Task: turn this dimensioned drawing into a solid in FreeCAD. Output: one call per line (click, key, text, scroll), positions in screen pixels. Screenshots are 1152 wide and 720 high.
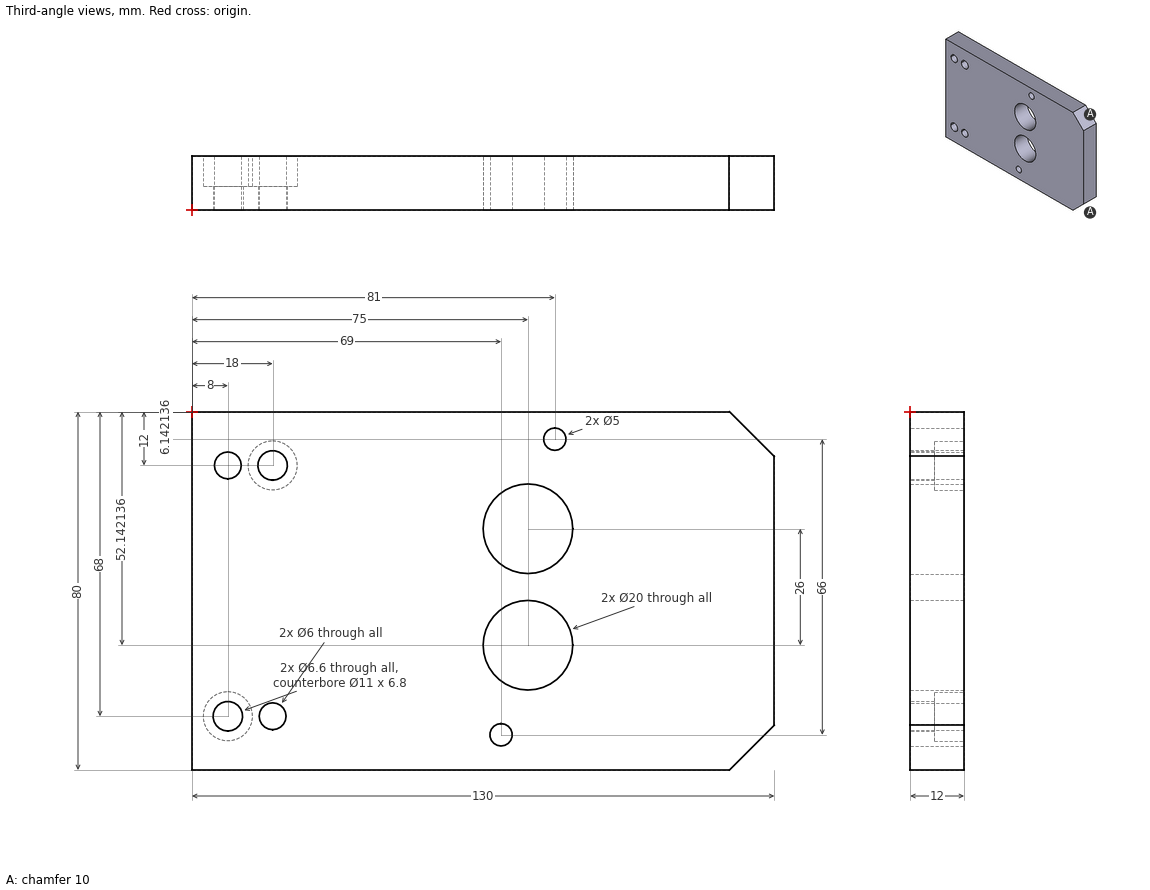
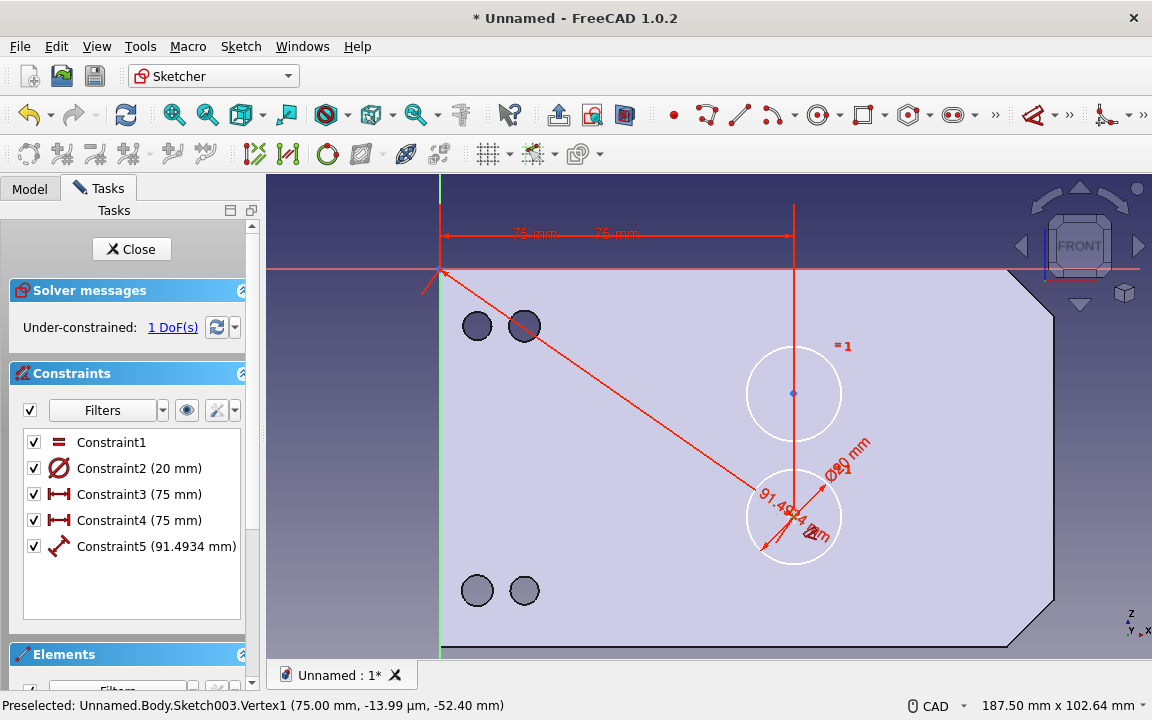
click(794, 394)
click(760, 456)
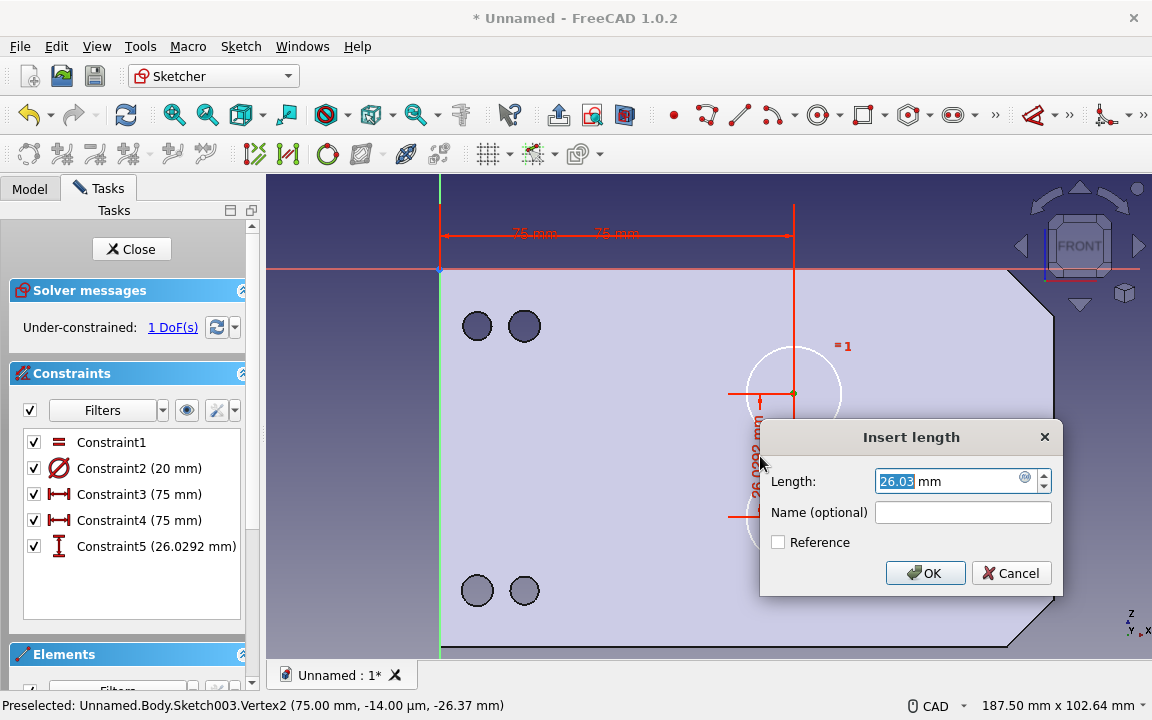
text(26)
key(Return)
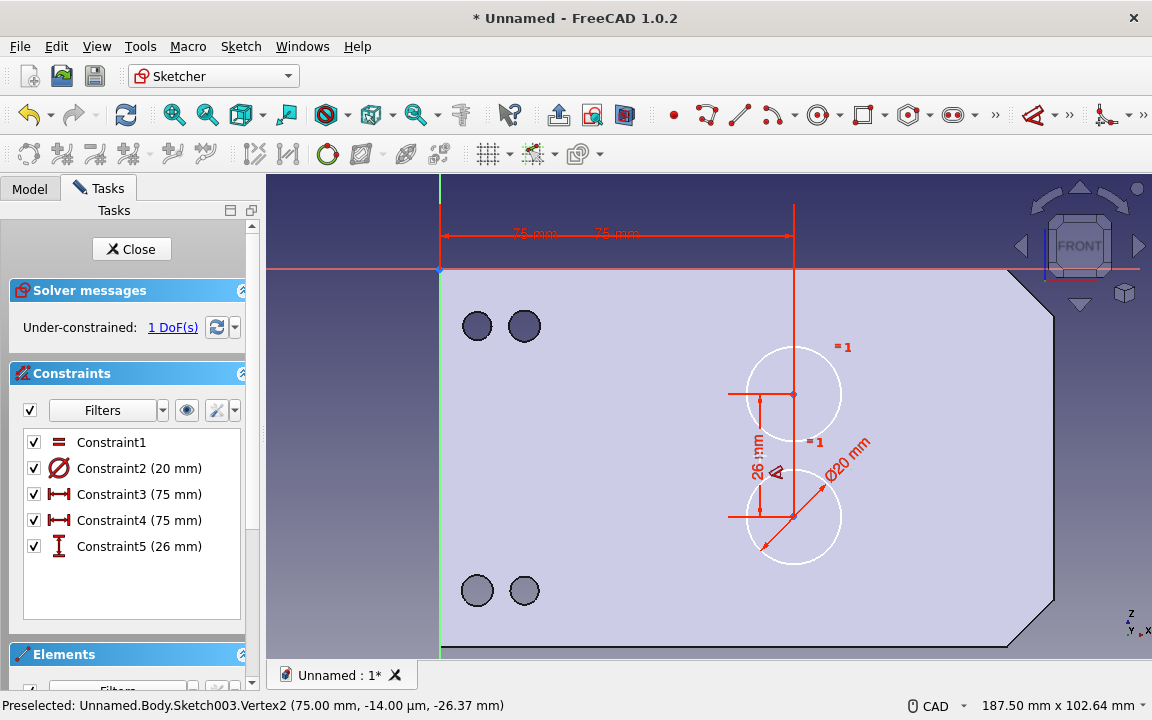
click(794, 517)
click(406, 393)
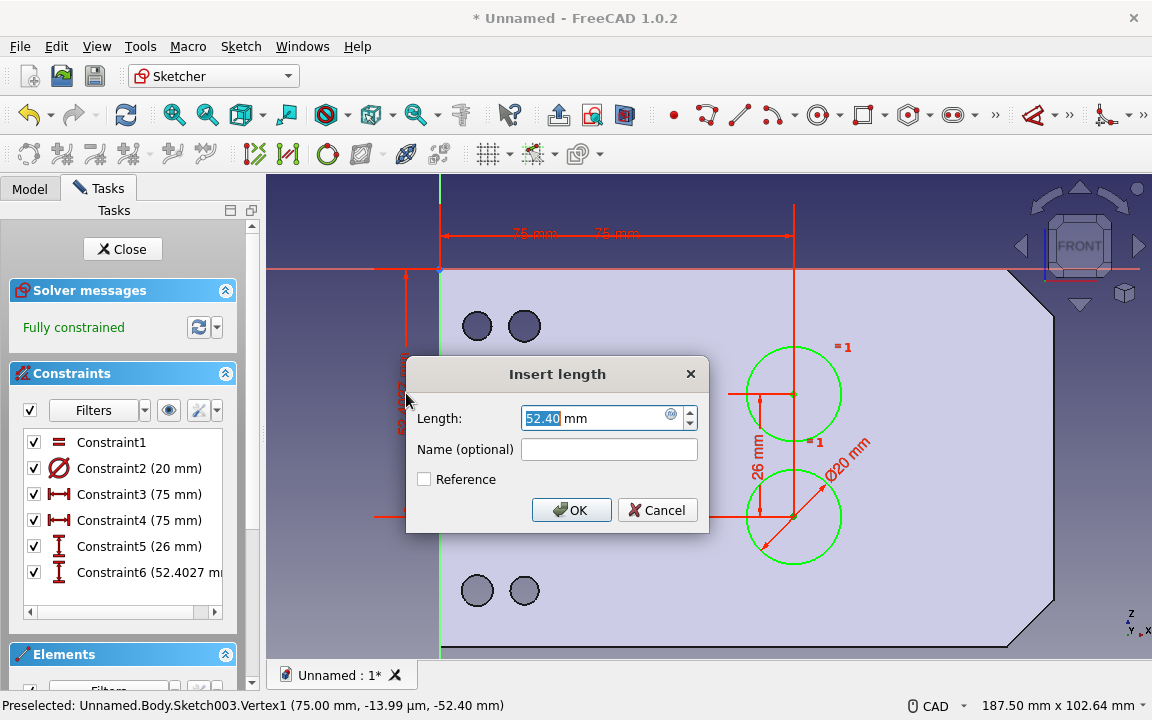
text(52.142136)
key(Return)
key(Escape)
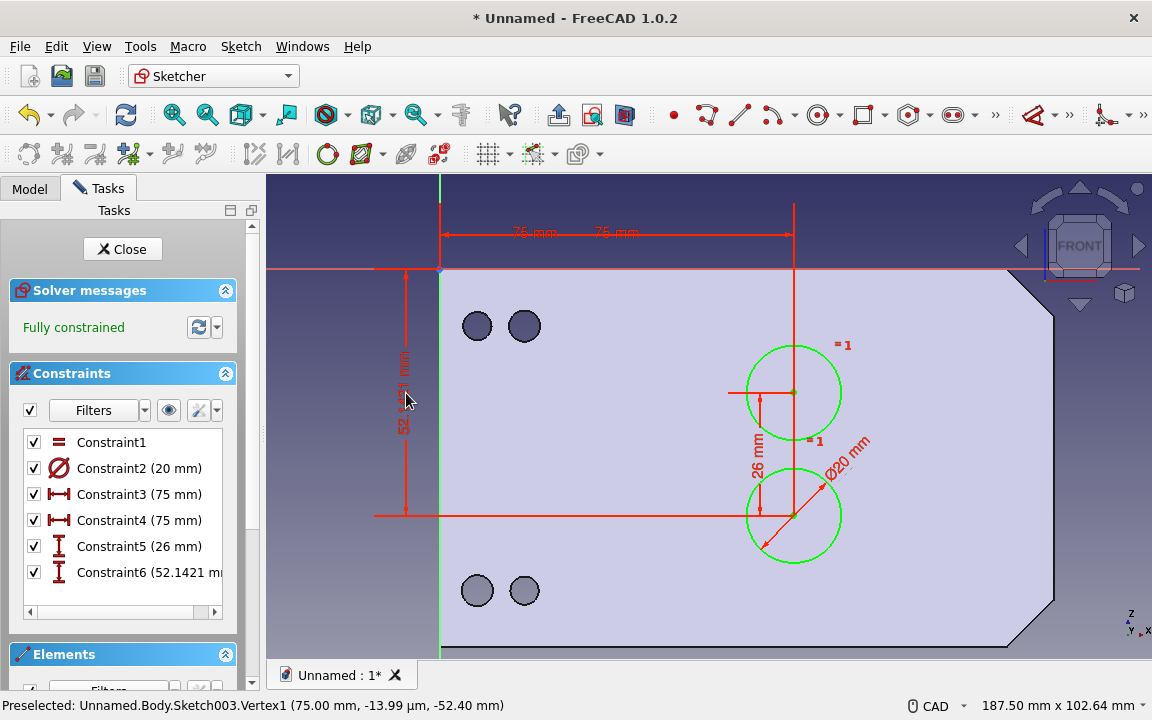
click(123, 249)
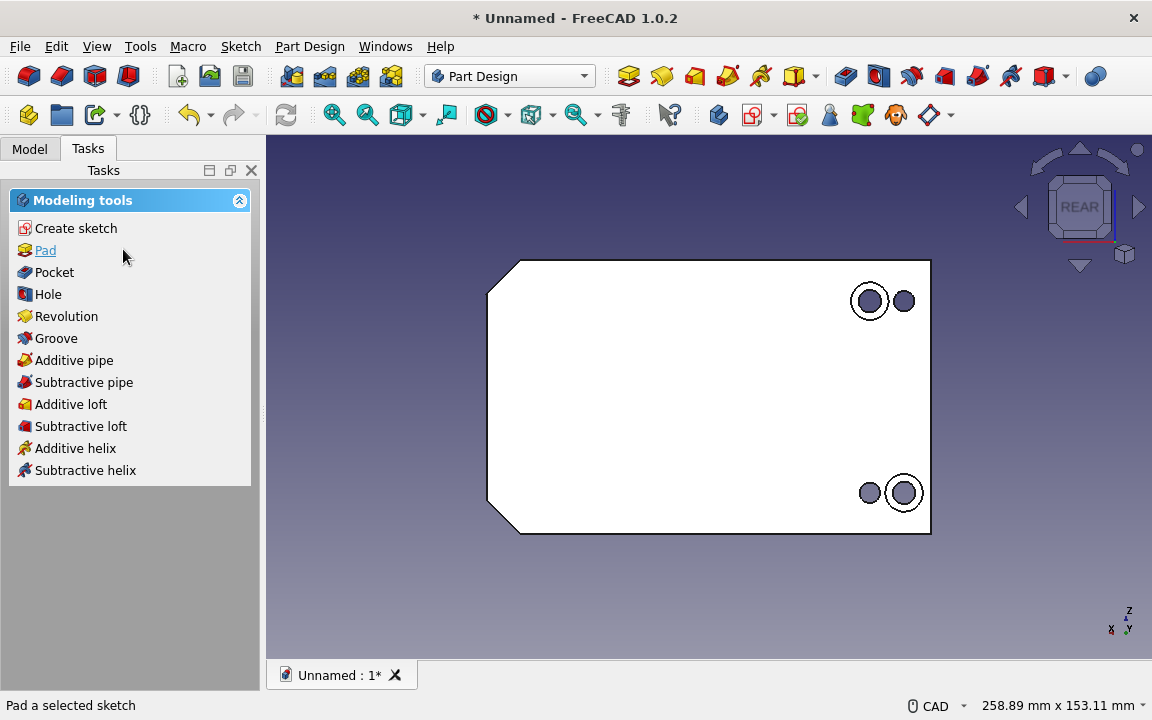
click(879, 76)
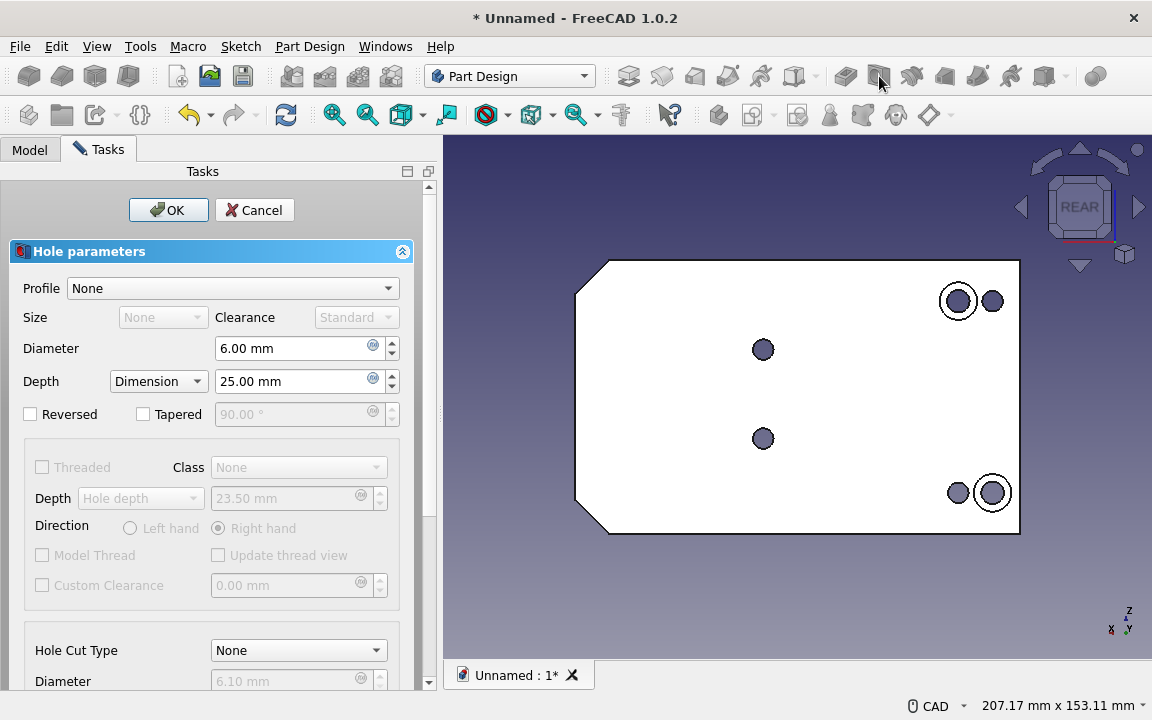
triple_click(300, 348)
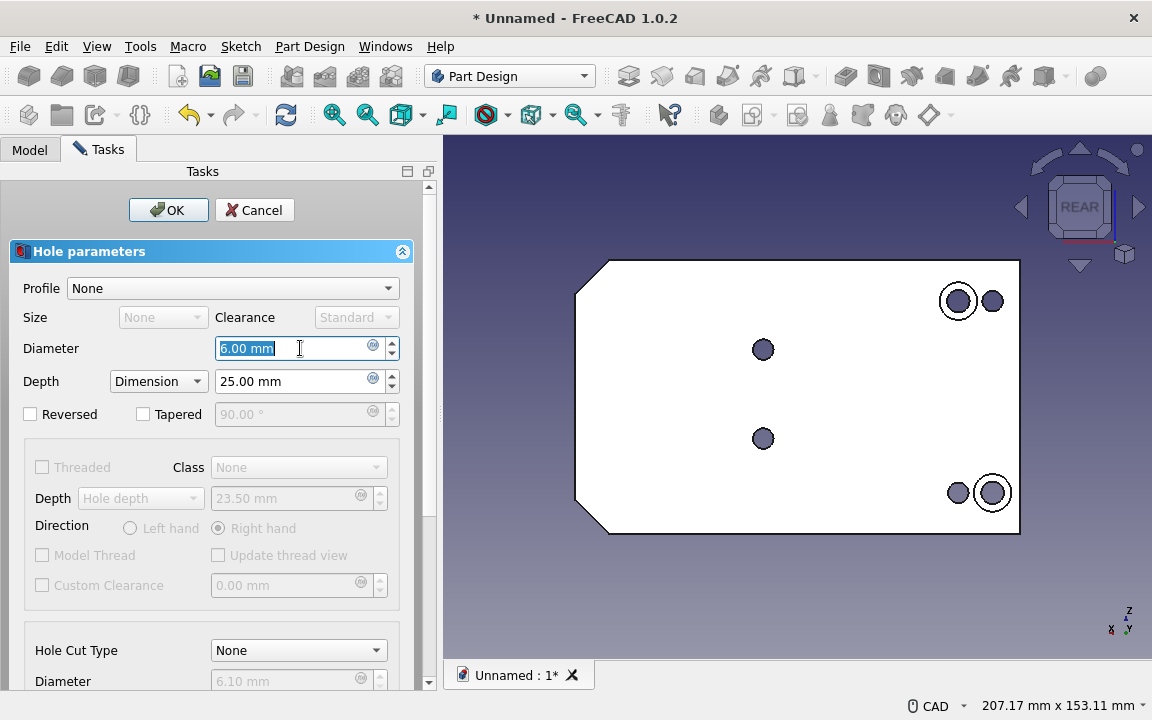
text(20)
key(Tab)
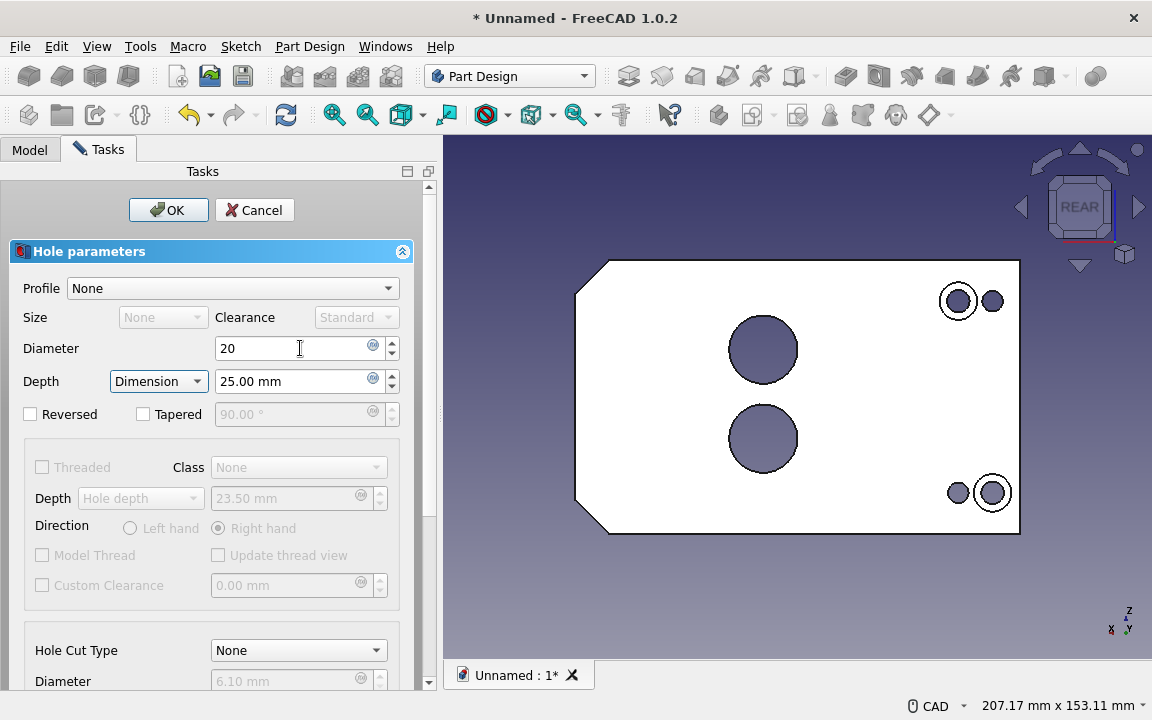
click(160, 382)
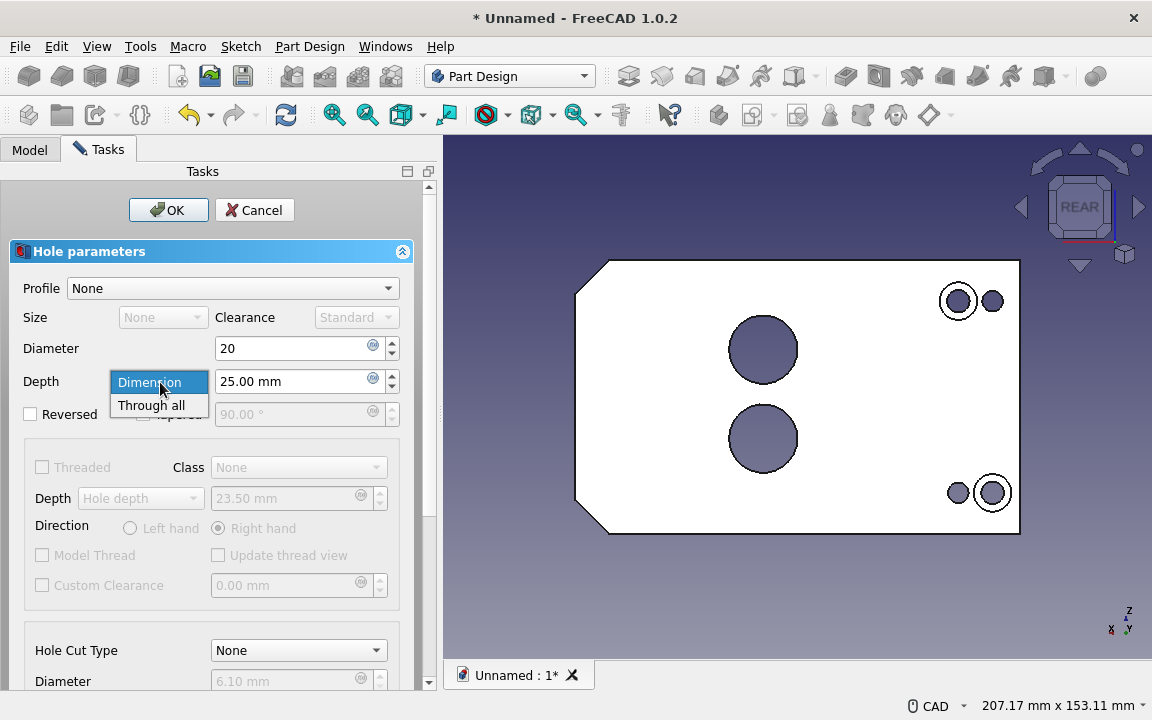
click(158, 406)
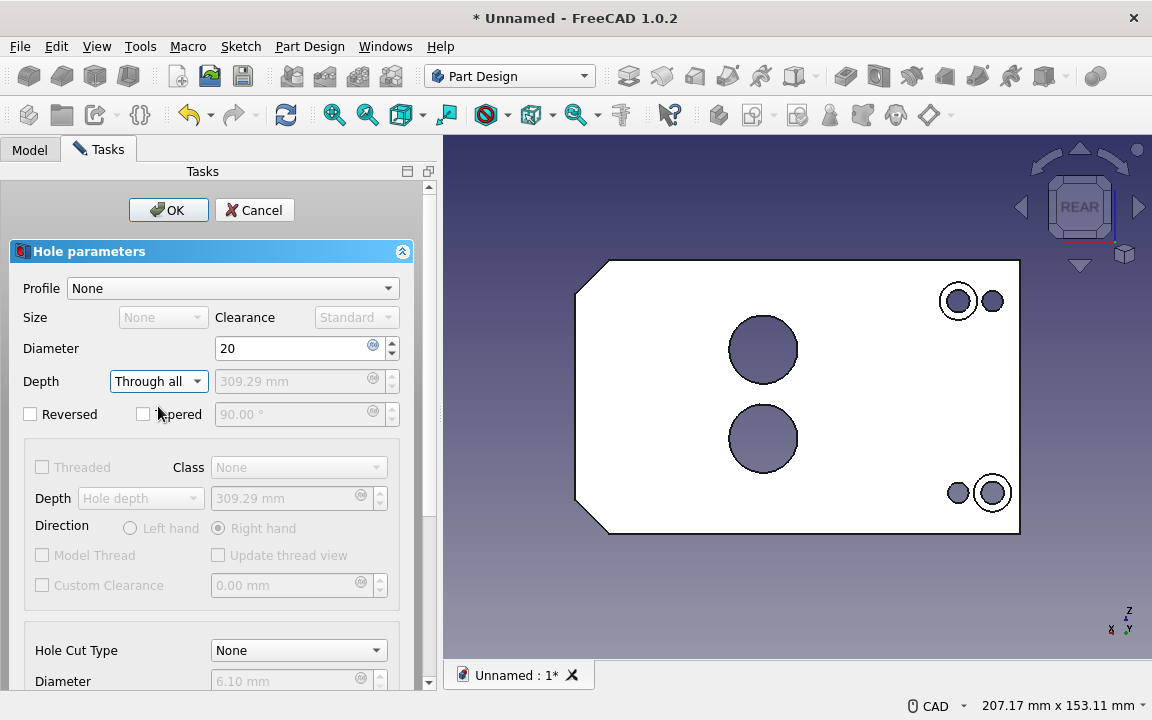
click(169, 210)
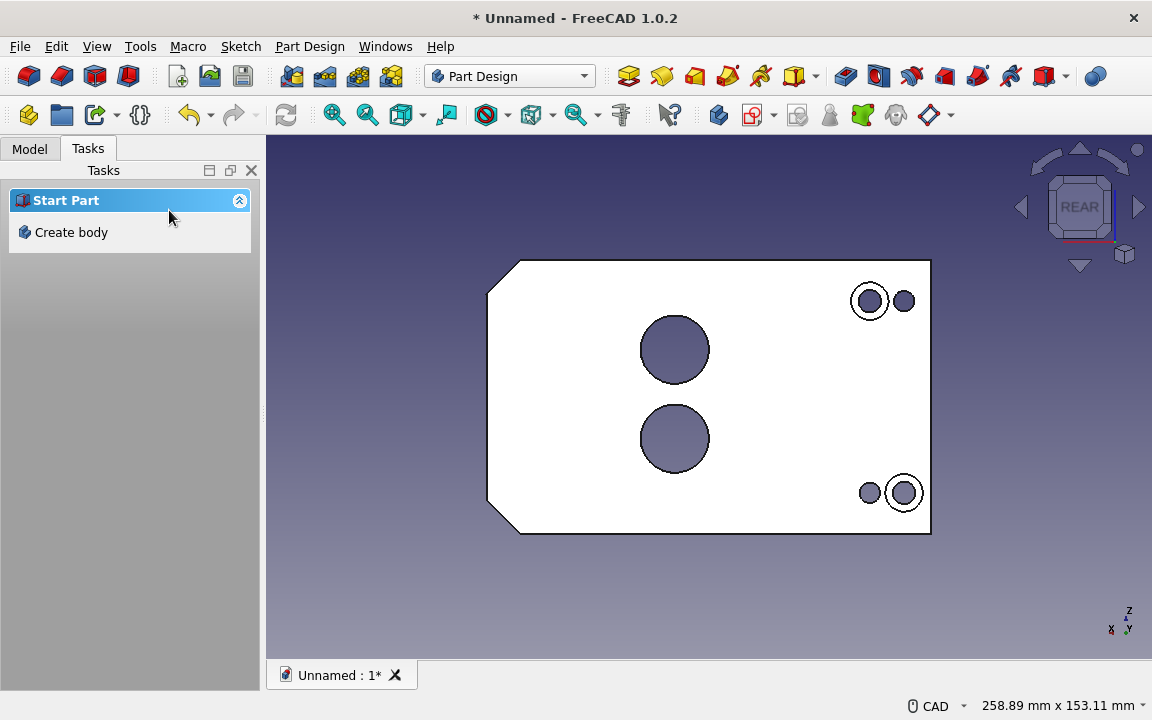
click(836, 396)